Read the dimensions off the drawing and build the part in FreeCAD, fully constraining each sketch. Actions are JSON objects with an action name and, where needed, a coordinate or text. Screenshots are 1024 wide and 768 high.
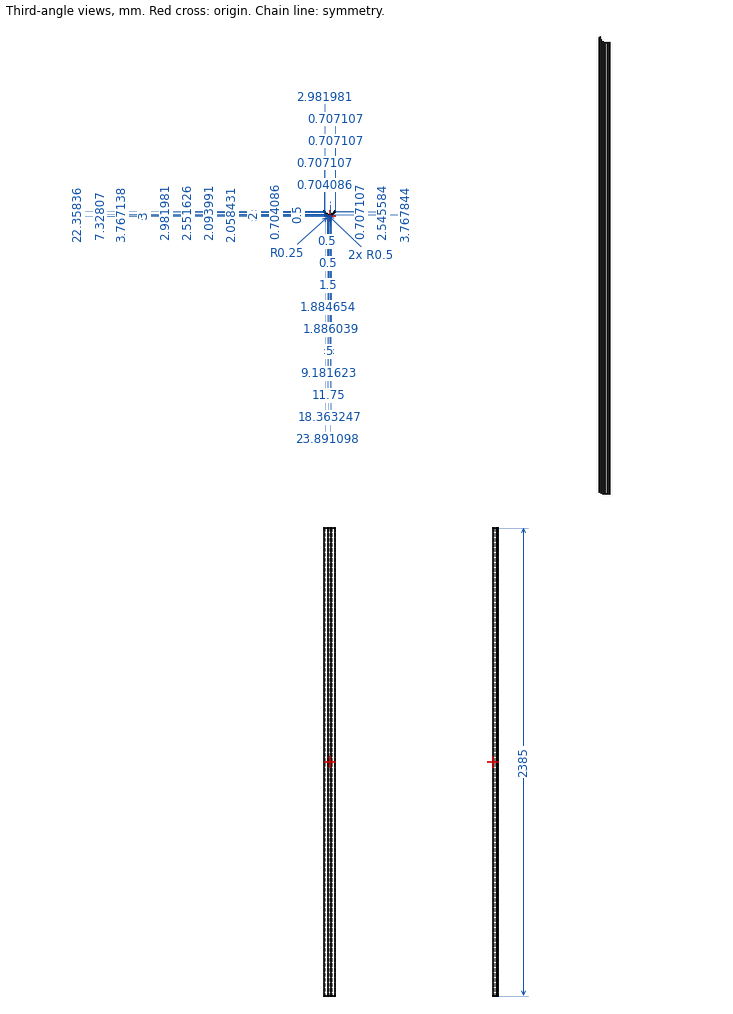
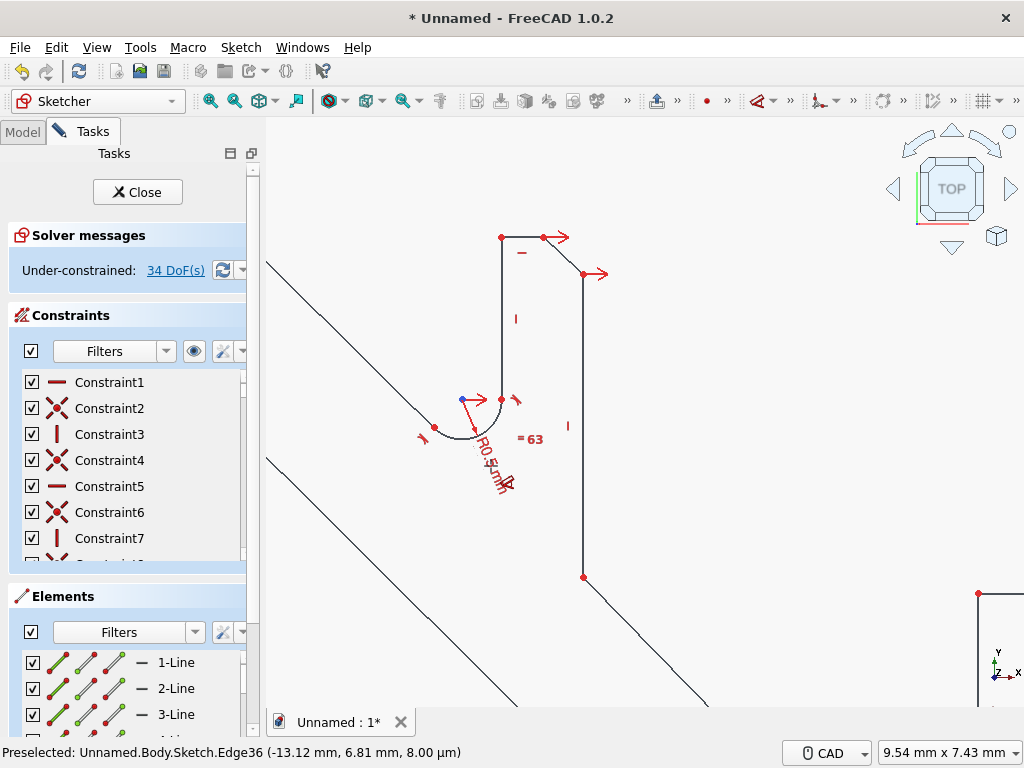
{"action": "scroll", "coordinate": [483, 444], "scroll_direction": "down", "scroll_amount": 12}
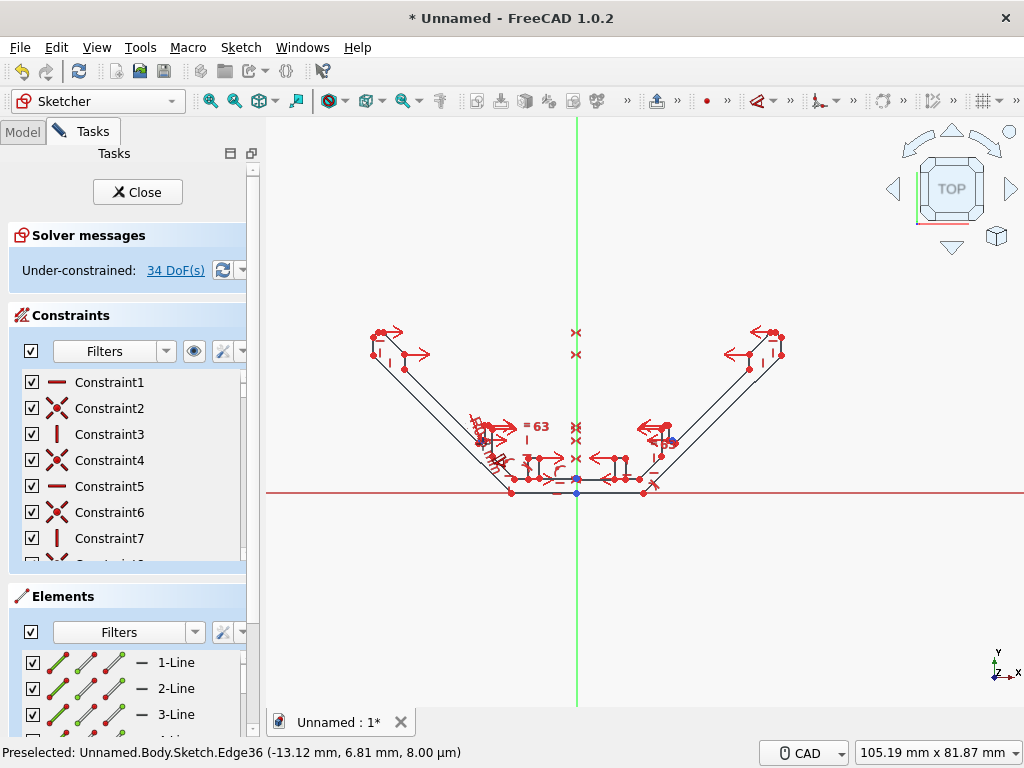
{"action": "scroll", "coordinate": [576, 480], "scroll_direction": "up", "scroll_amount": 16}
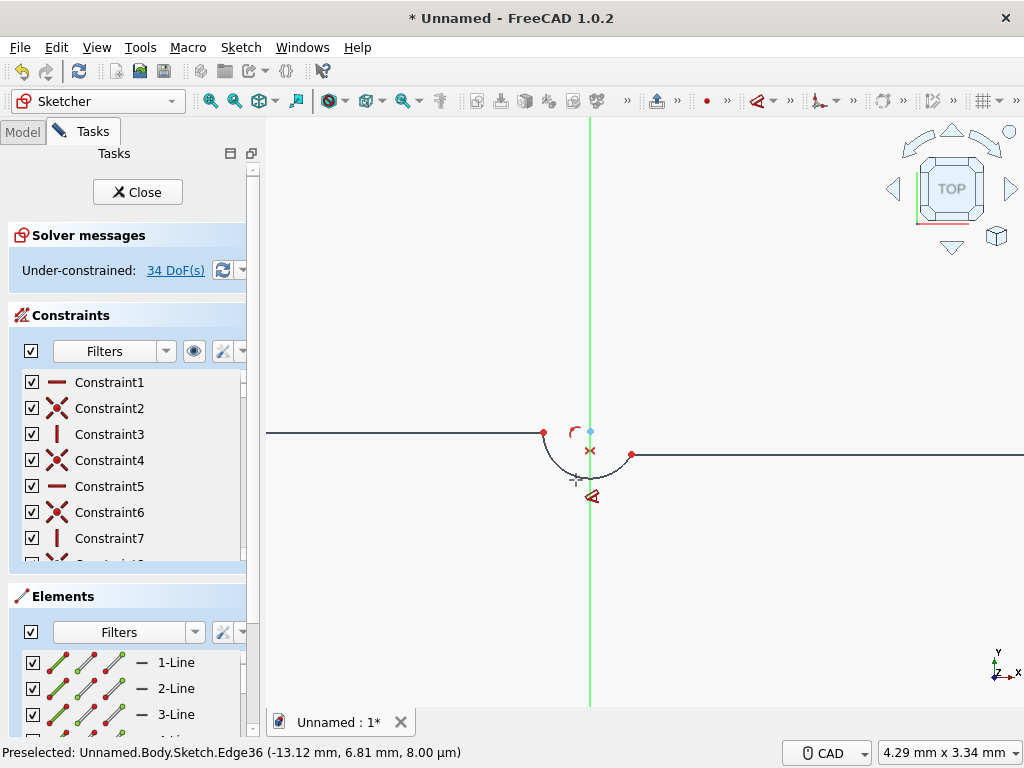
{"action": "left_click", "coordinate": [558, 466]}
{"action": "left_click", "coordinate": [536, 489]}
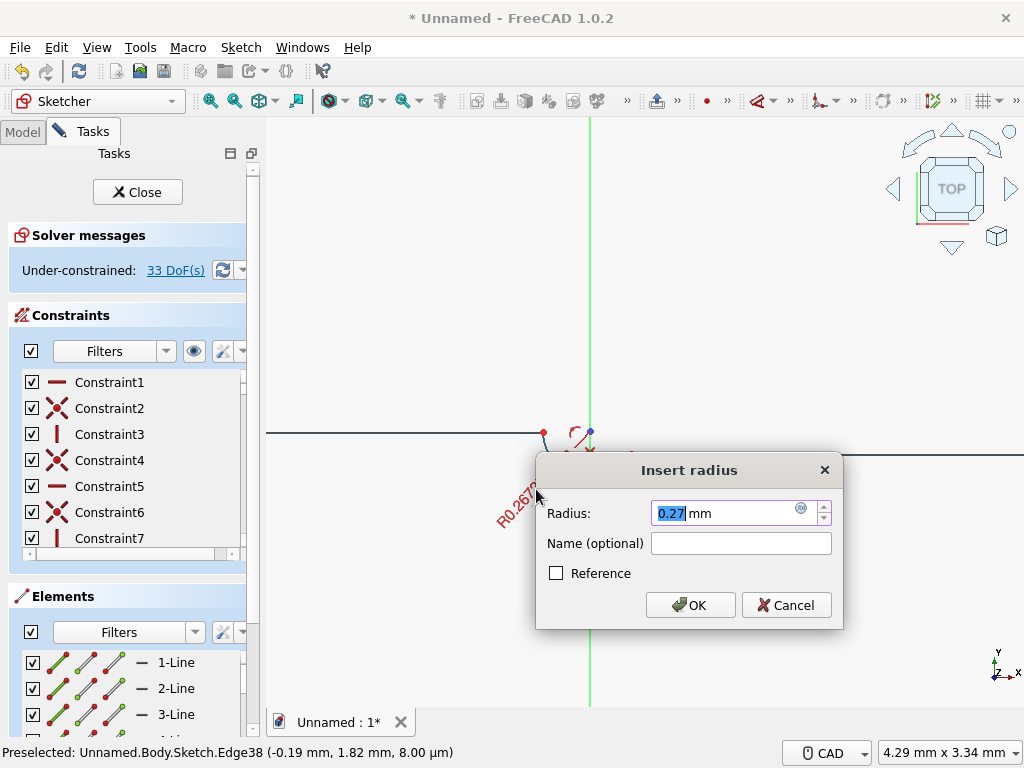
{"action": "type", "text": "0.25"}
{"action": "key", "text": "Return"}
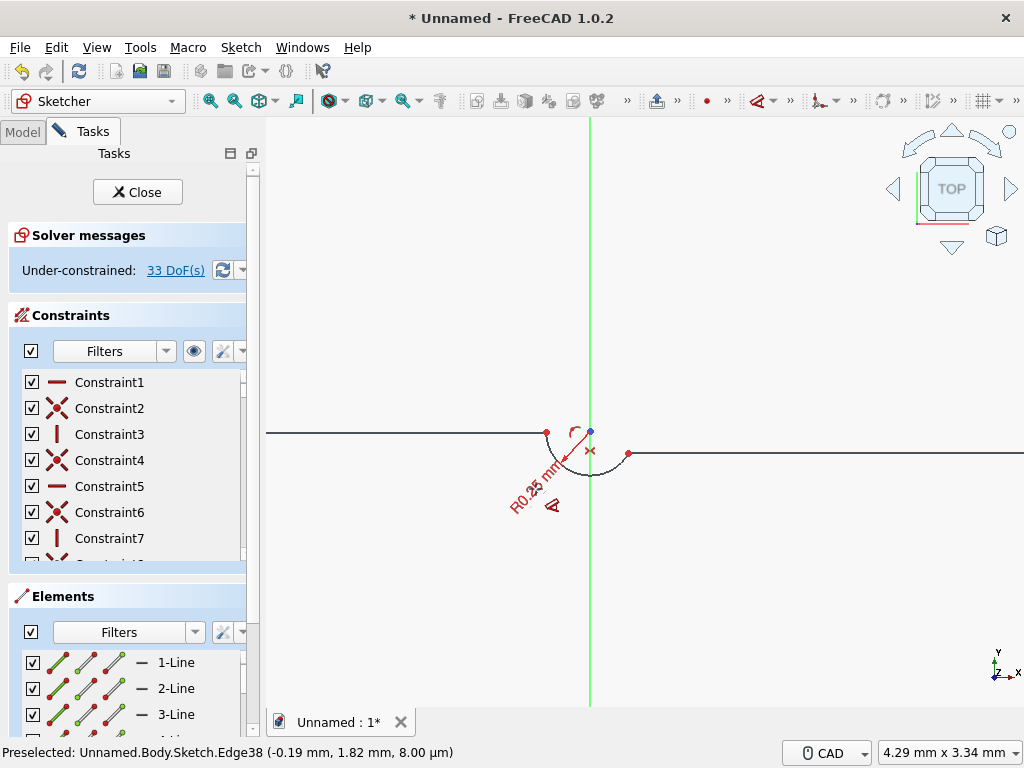
{"action": "scroll", "coordinate": [576, 496], "scroll_direction": "down", "scroll_amount": 15}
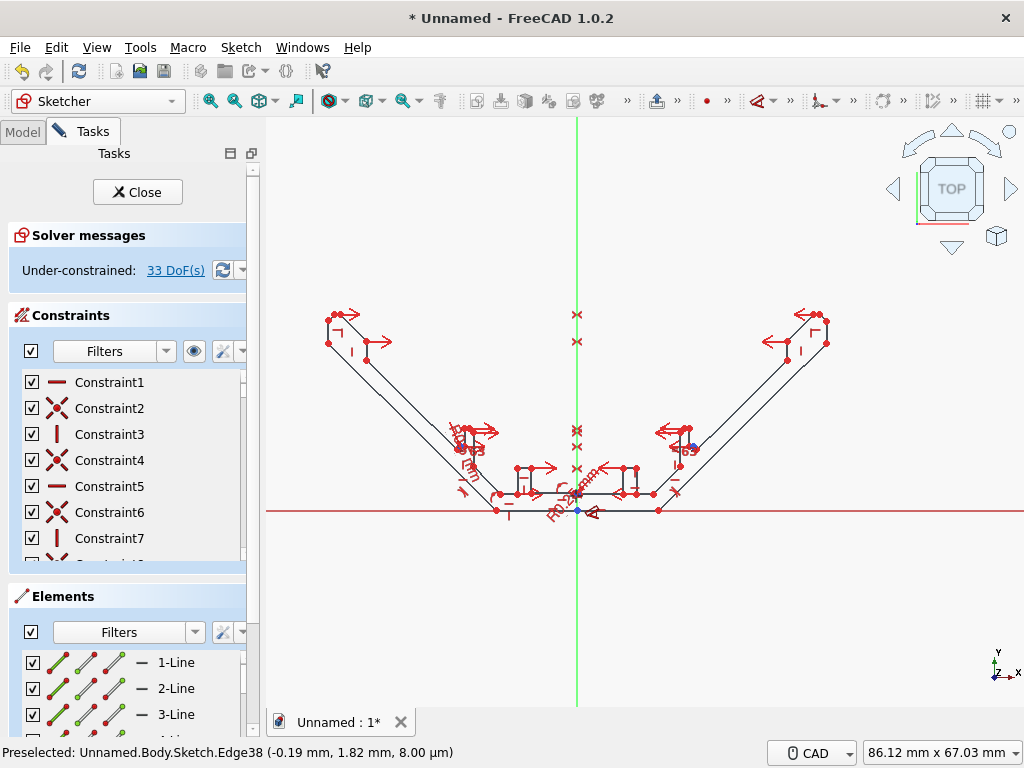
{"action": "scroll", "coordinate": [566, 493], "scroll_direction": "up", "scroll_amount": 3}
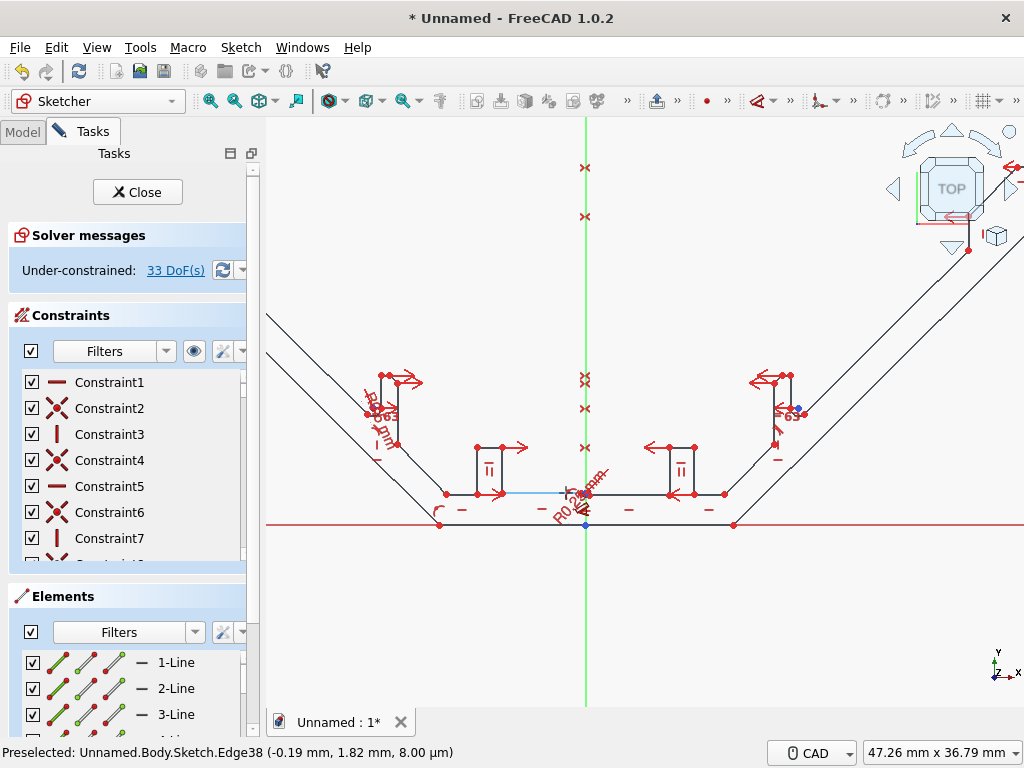
{"action": "left_click", "coordinate": [566, 493]}
{"action": "left_click", "coordinate": [542, 459]}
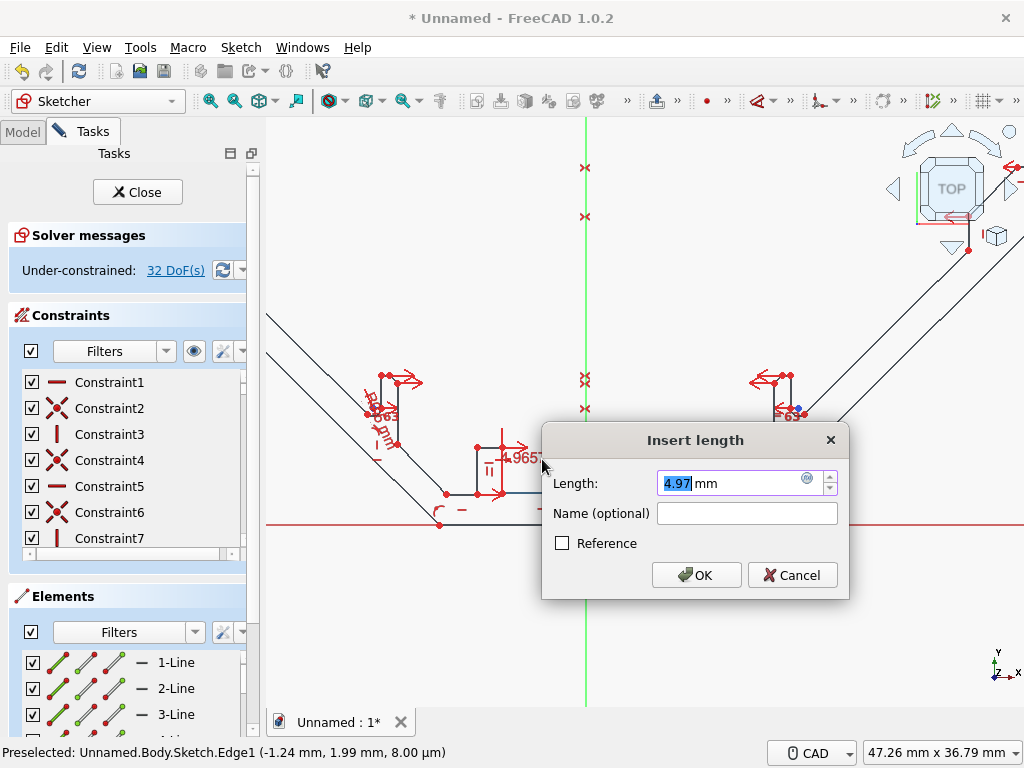
{"action": "type", "text": "5"}
{"action": "key", "text": "Return"}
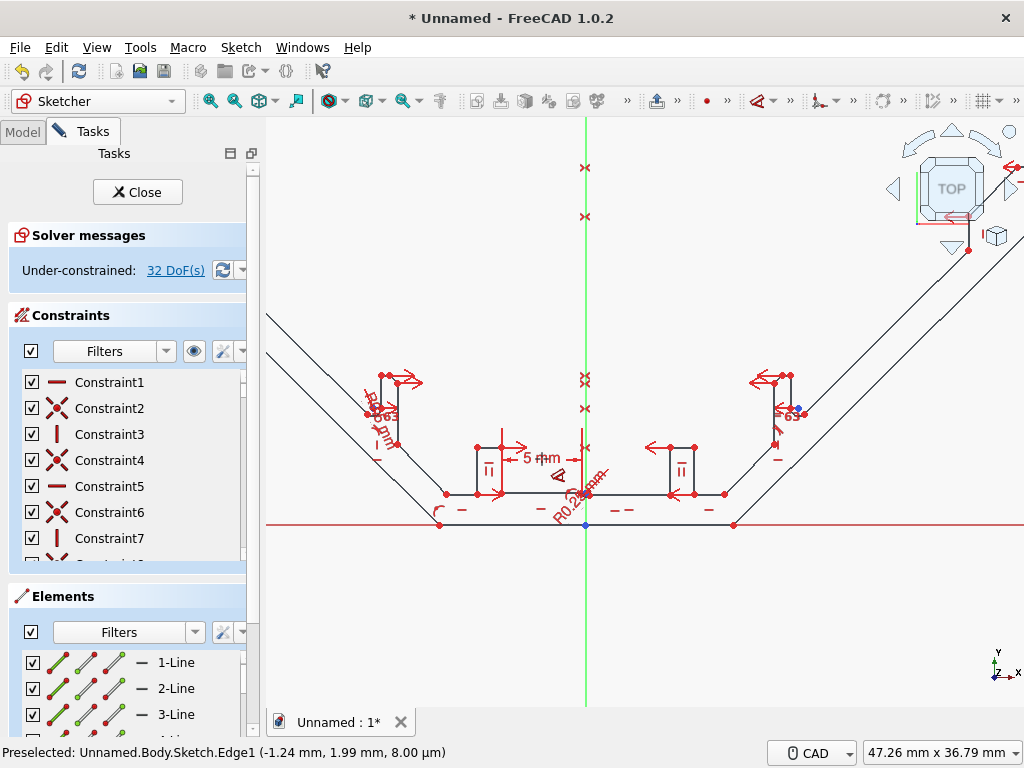
{"action": "left_click", "coordinate": [502, 480]}
{"action": "left_click", "coordinate": [444, 470]}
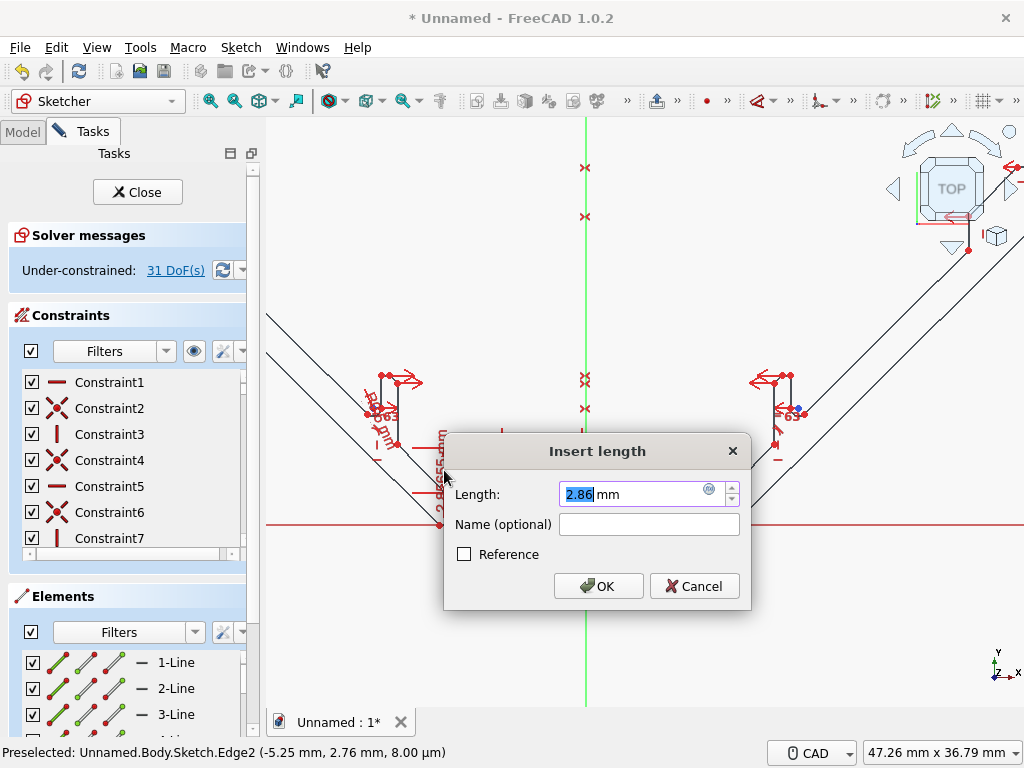
{"action": "type", "text": "3"}
{"action": "key", "text": "Return"}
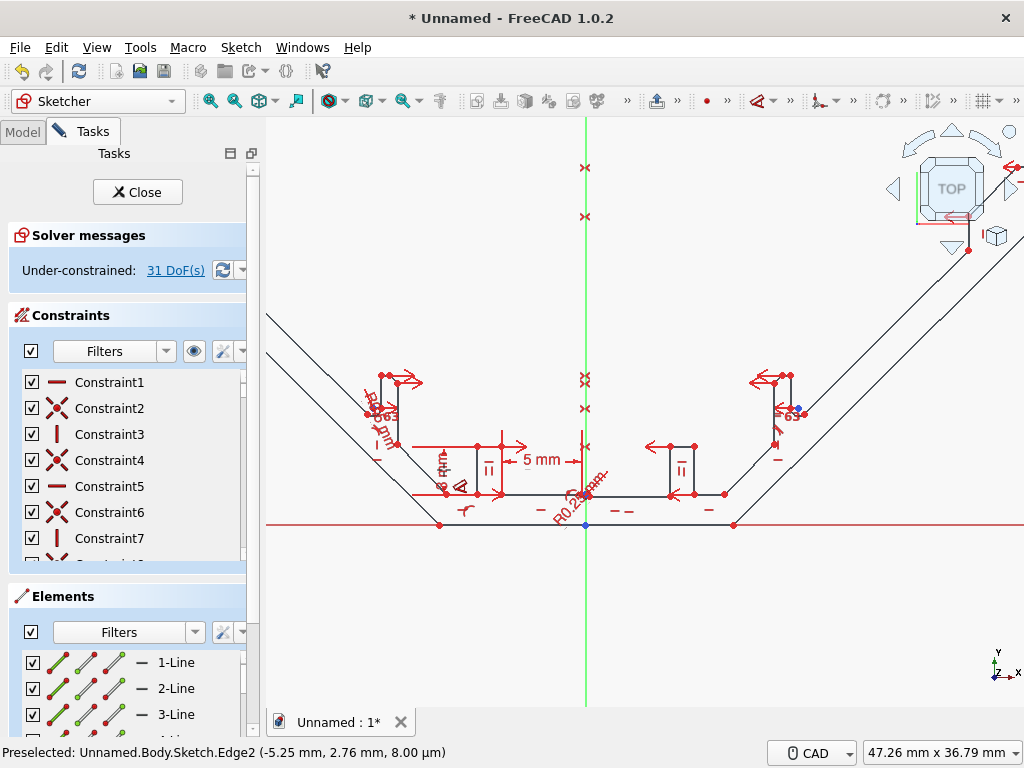
{"action": "left_click", "coordinate": [477, 461]}
{"action": "left_click", "coordinate": [371, 482]}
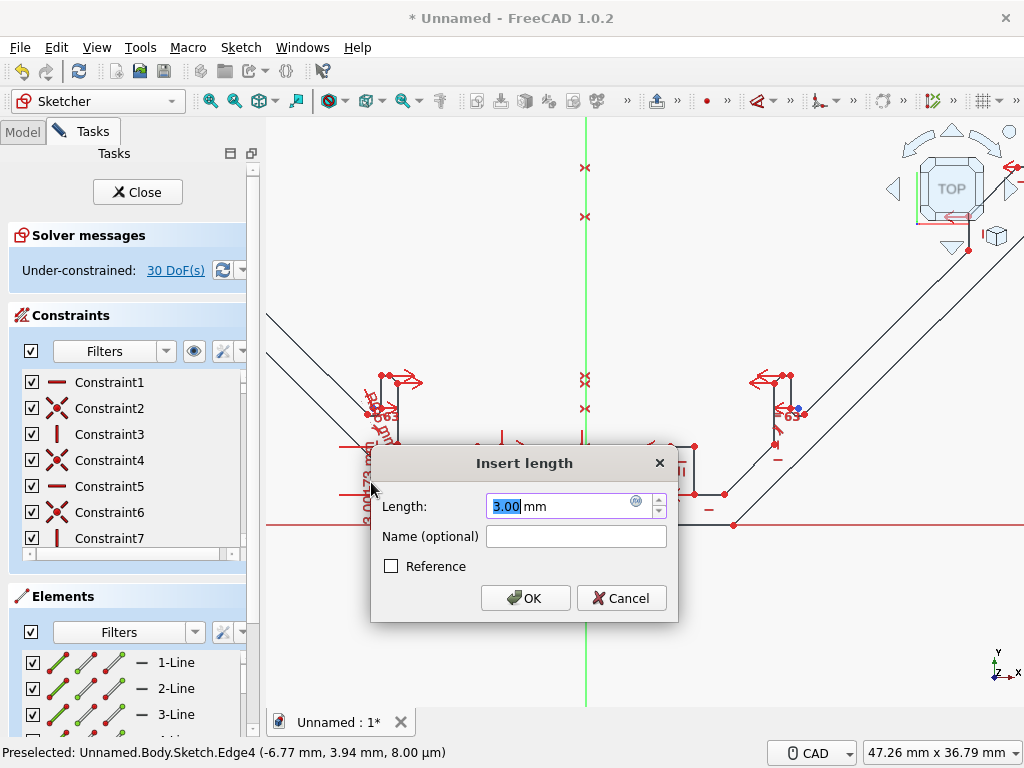
{"action": "type", "text": "3"}
{"action": "key", "text": "Return"}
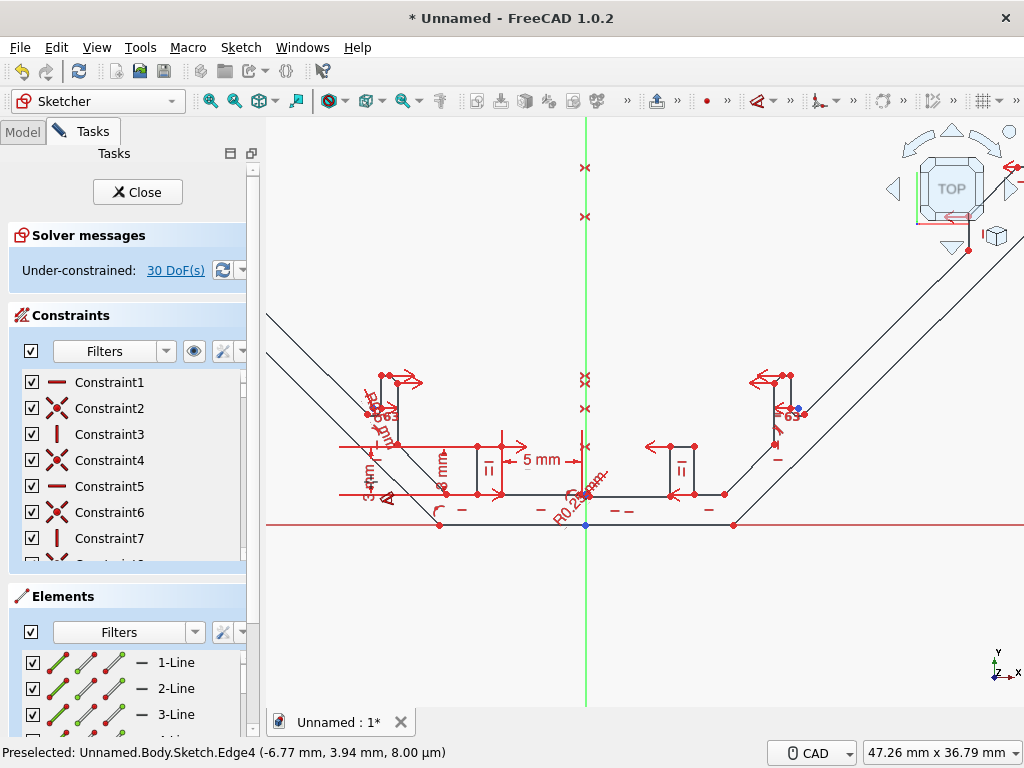
{"action": "left_click", "coordinate": [670, 462]}
{"action": "left_click", "coordinate": [636, 472]}